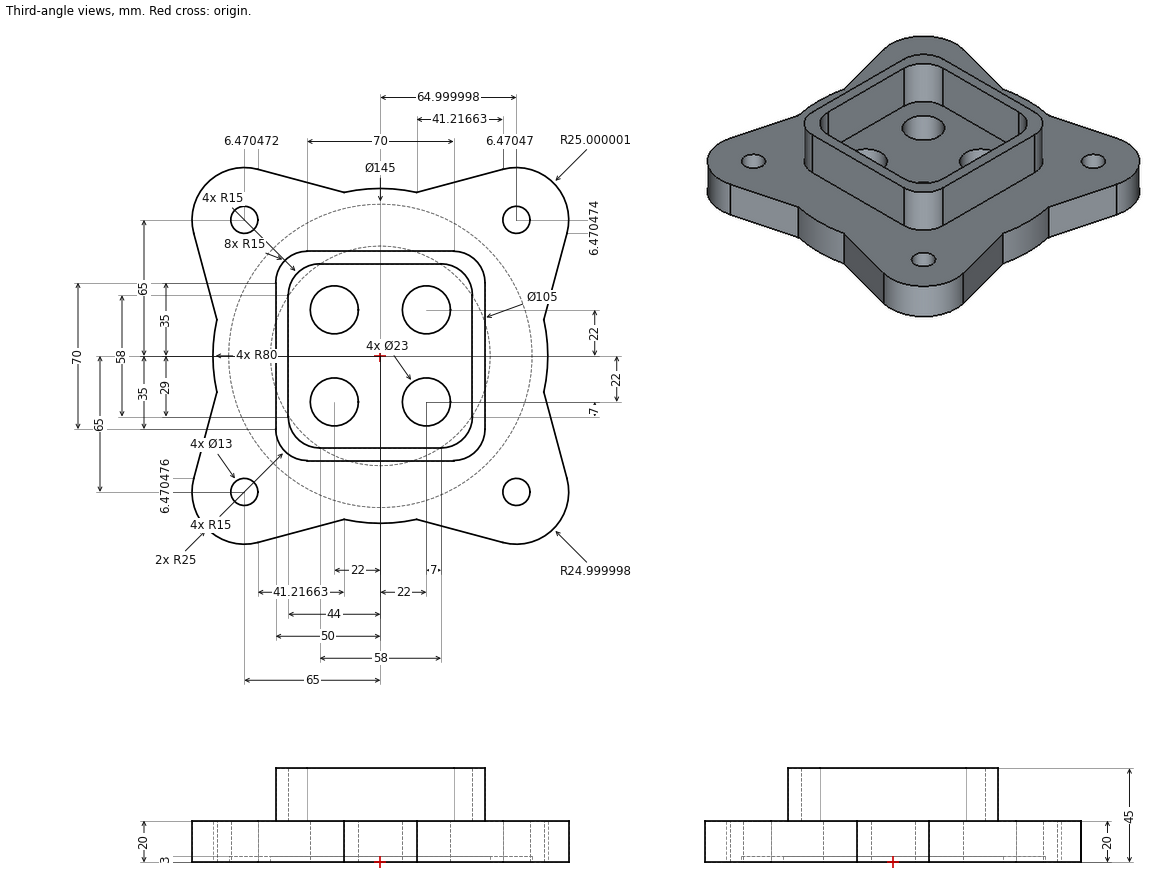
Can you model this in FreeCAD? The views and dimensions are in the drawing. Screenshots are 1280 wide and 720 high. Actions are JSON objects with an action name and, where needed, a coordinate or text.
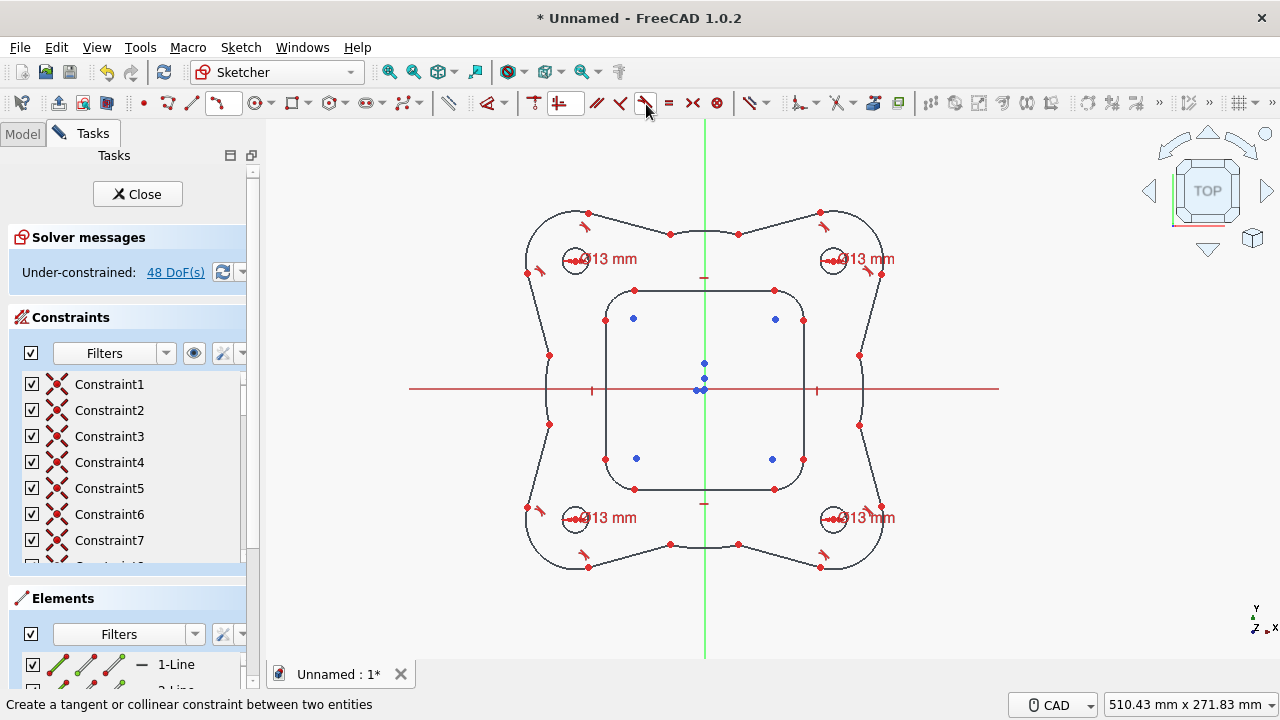
{"action": "left_click", "coordinate": [606, 418]}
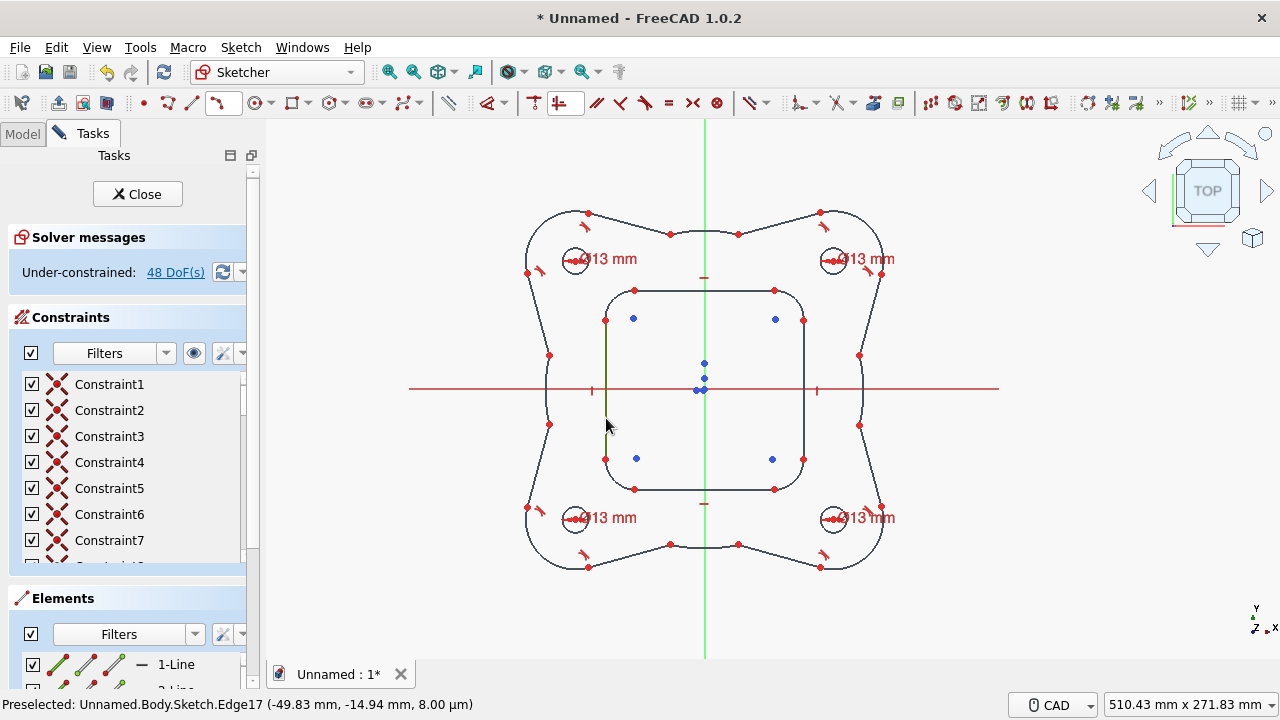
{"action": "left_click", "coordinate": [621, 294]}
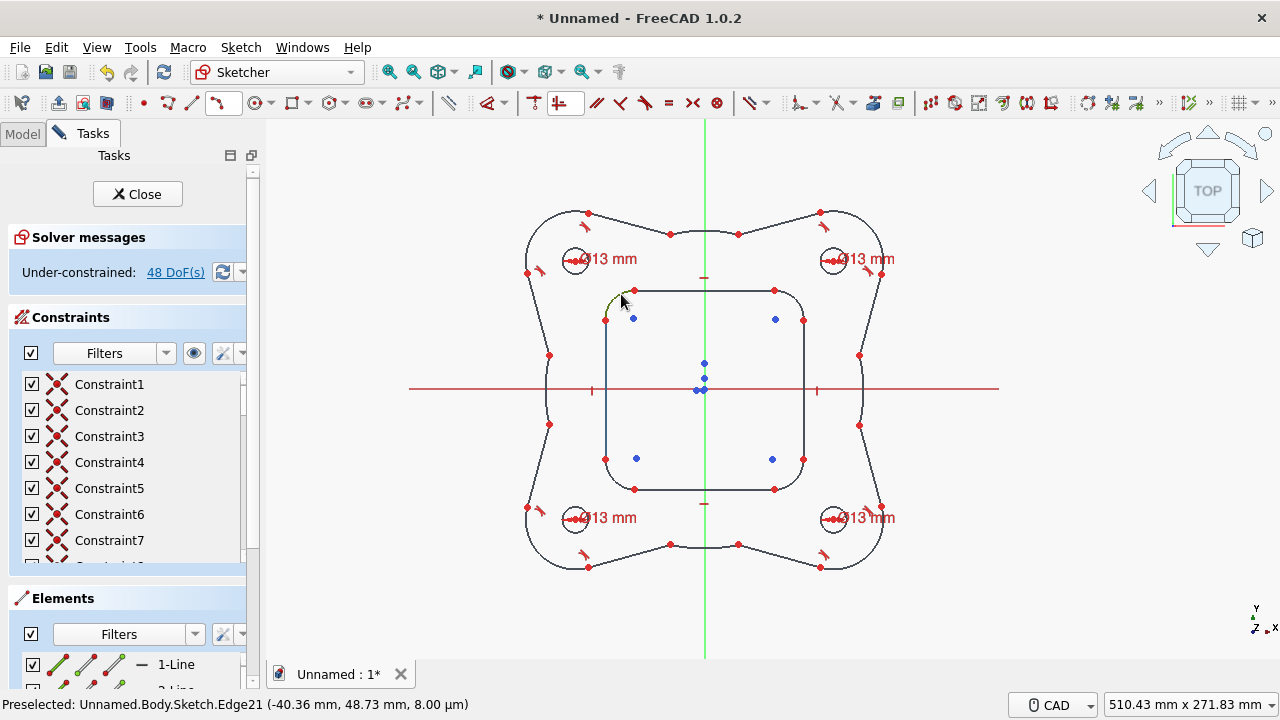
{"action": "left_click", "coordinate": [646, 104]}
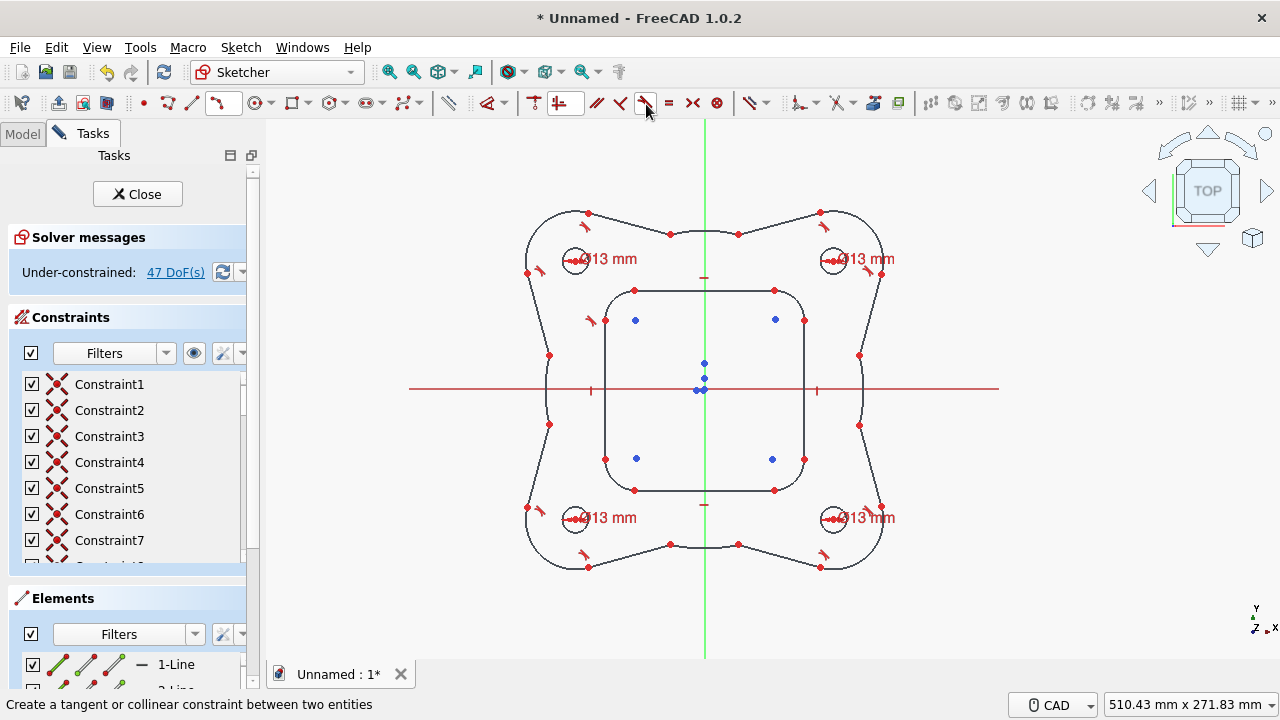
{"action": "left_click", "coordinate": [605, 418]}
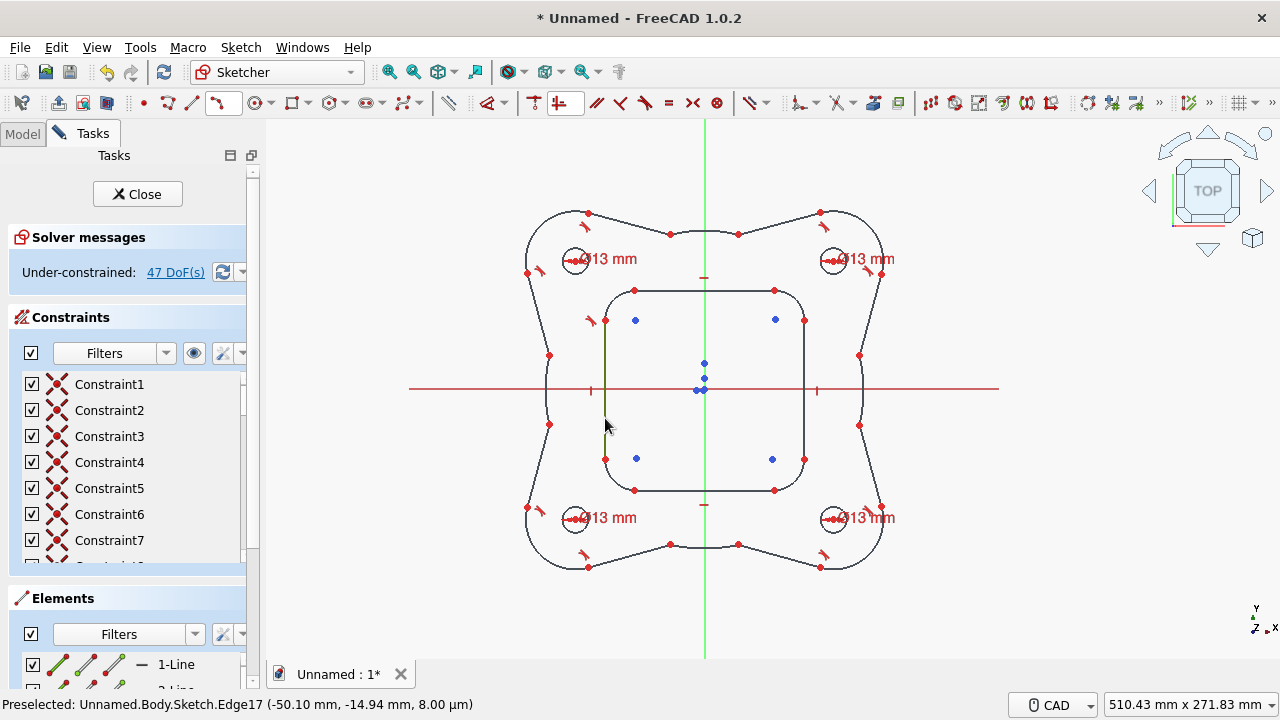
{"action": "left_click", "coordinate": [609, 473]}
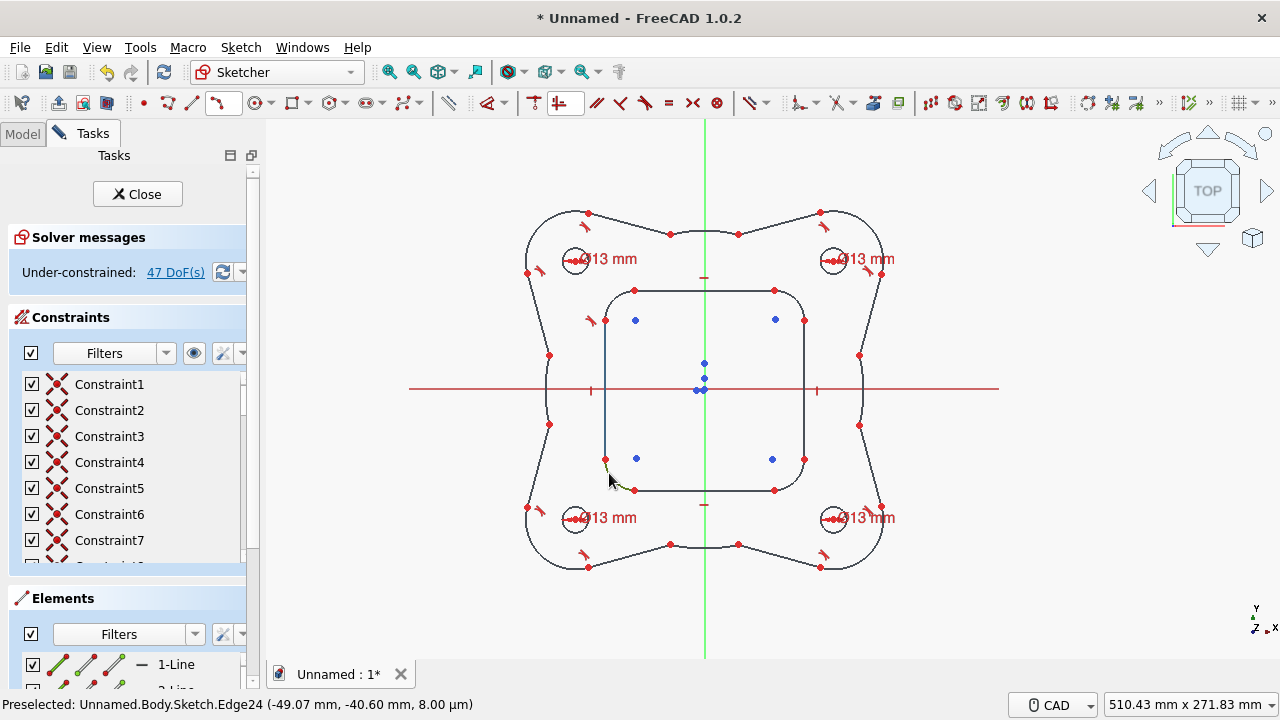
{"action": "left_click", "coordinate": [646, 104]}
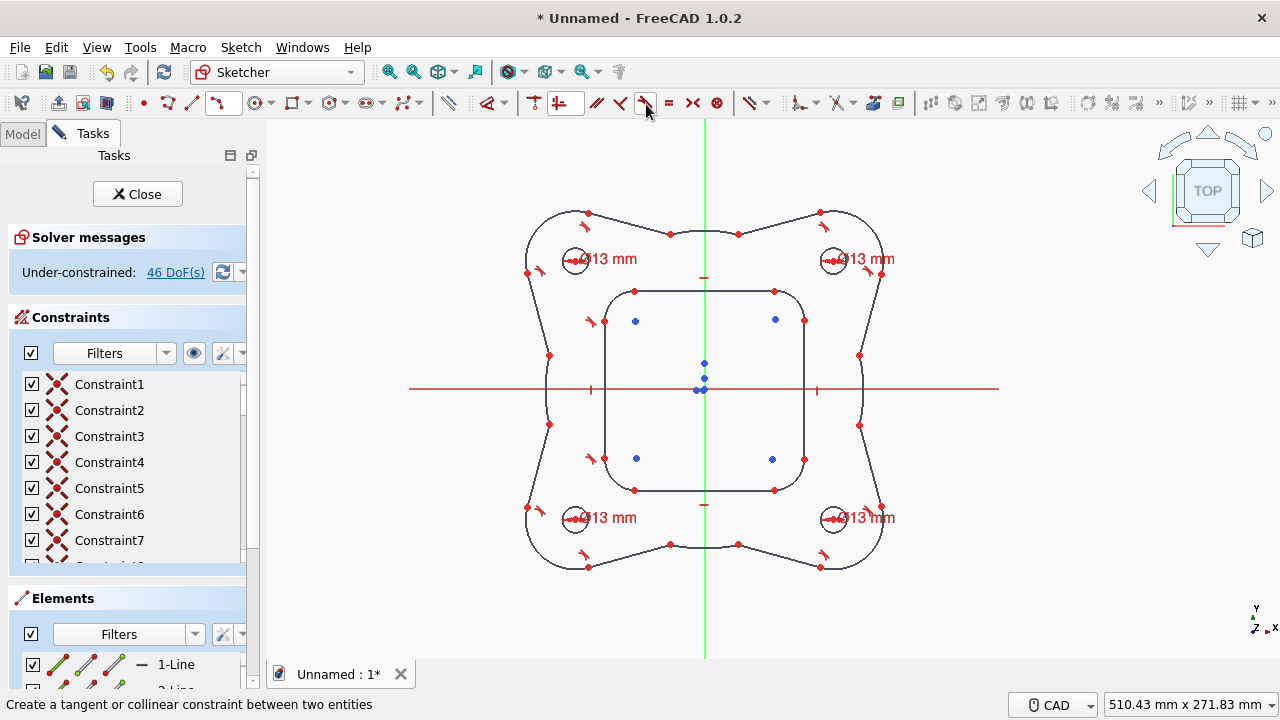
{"action": "left_click", "coordinate": [677, 291]}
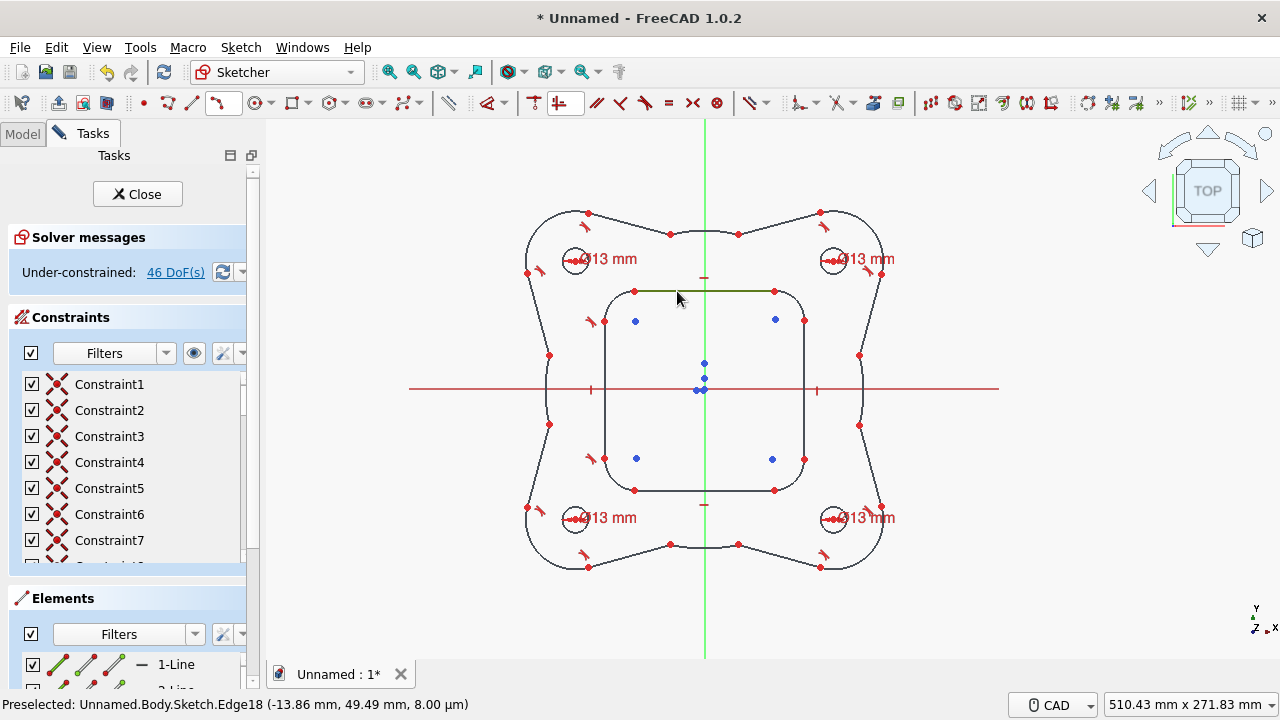
{"action": "left_click", "coordinate": [621, 294]}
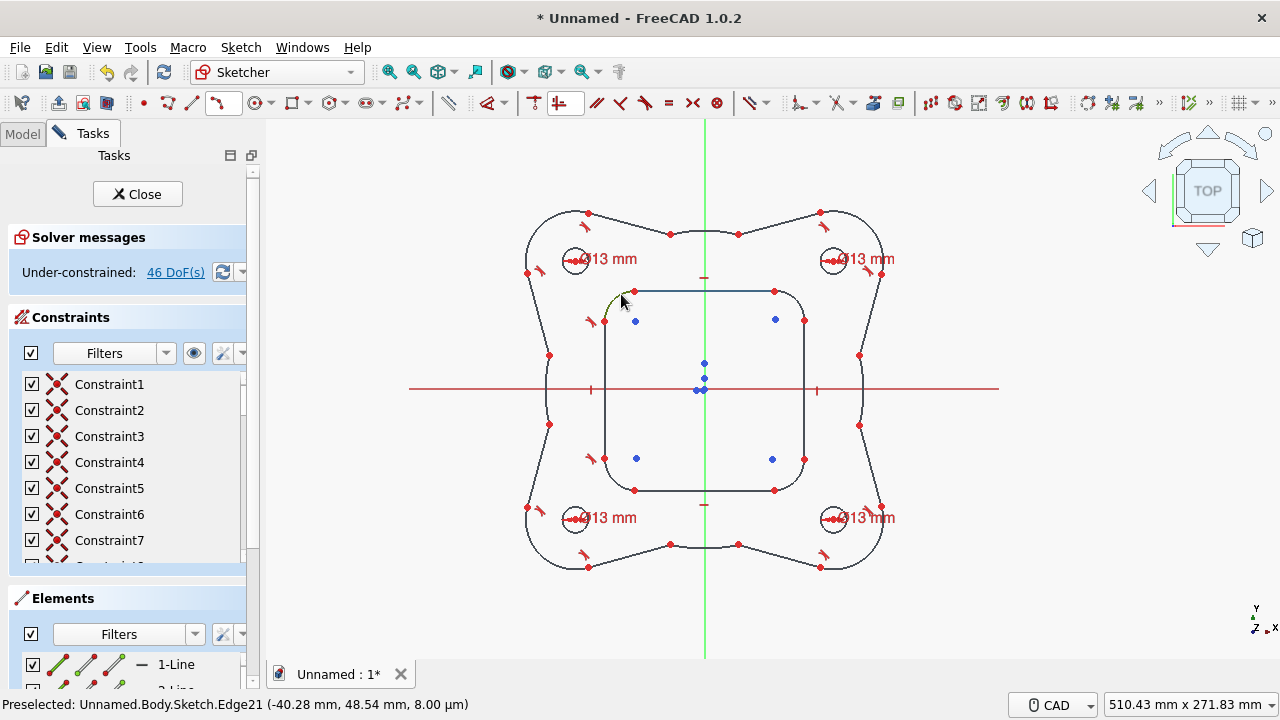
{"action": "key", "text": "t"}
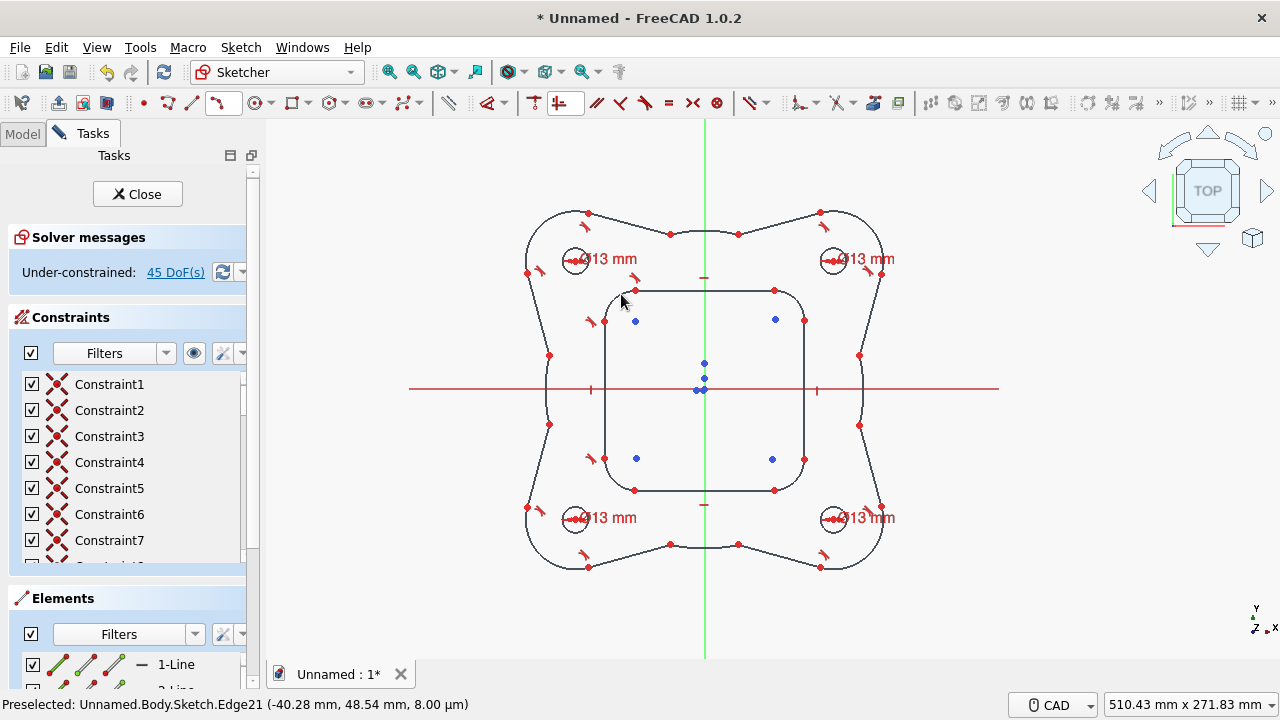
{"action": "left_click", "coordinate": [677, 291]}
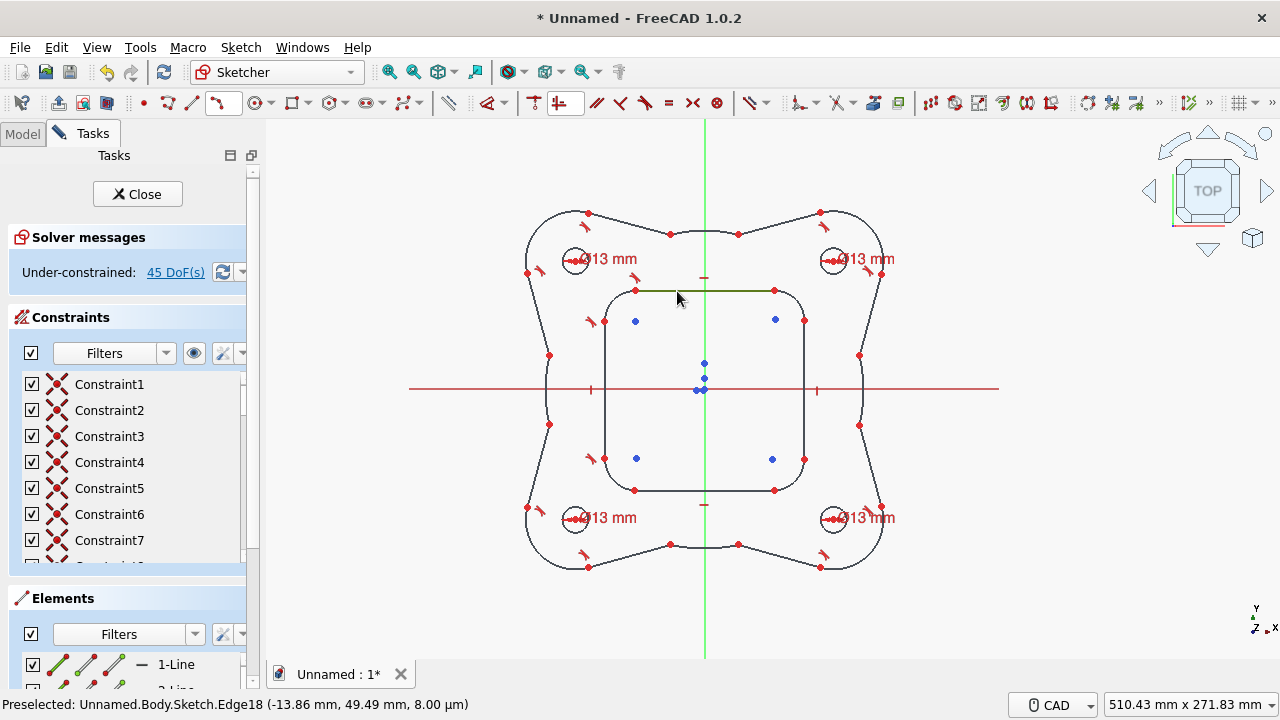
{"action": "left_click", "coordinate": [801, 307]}